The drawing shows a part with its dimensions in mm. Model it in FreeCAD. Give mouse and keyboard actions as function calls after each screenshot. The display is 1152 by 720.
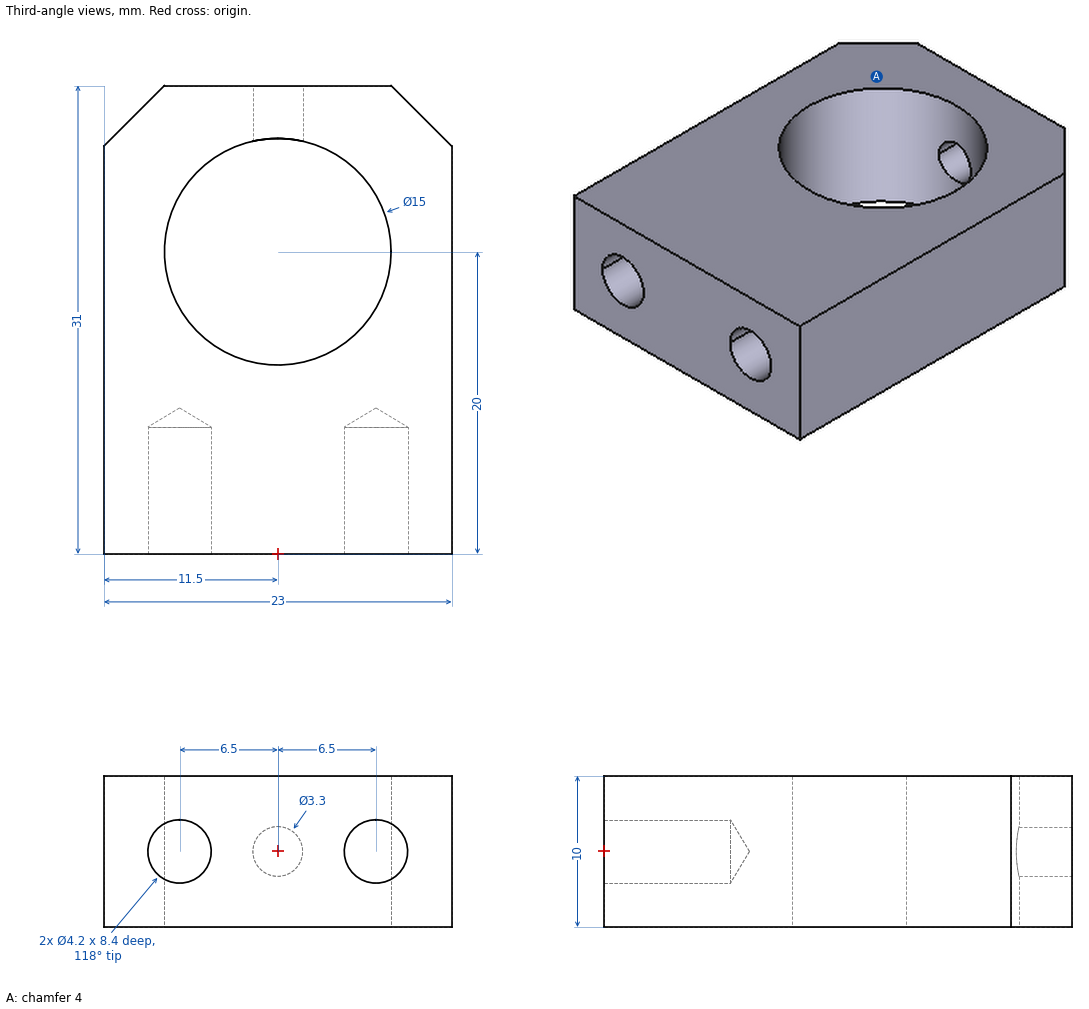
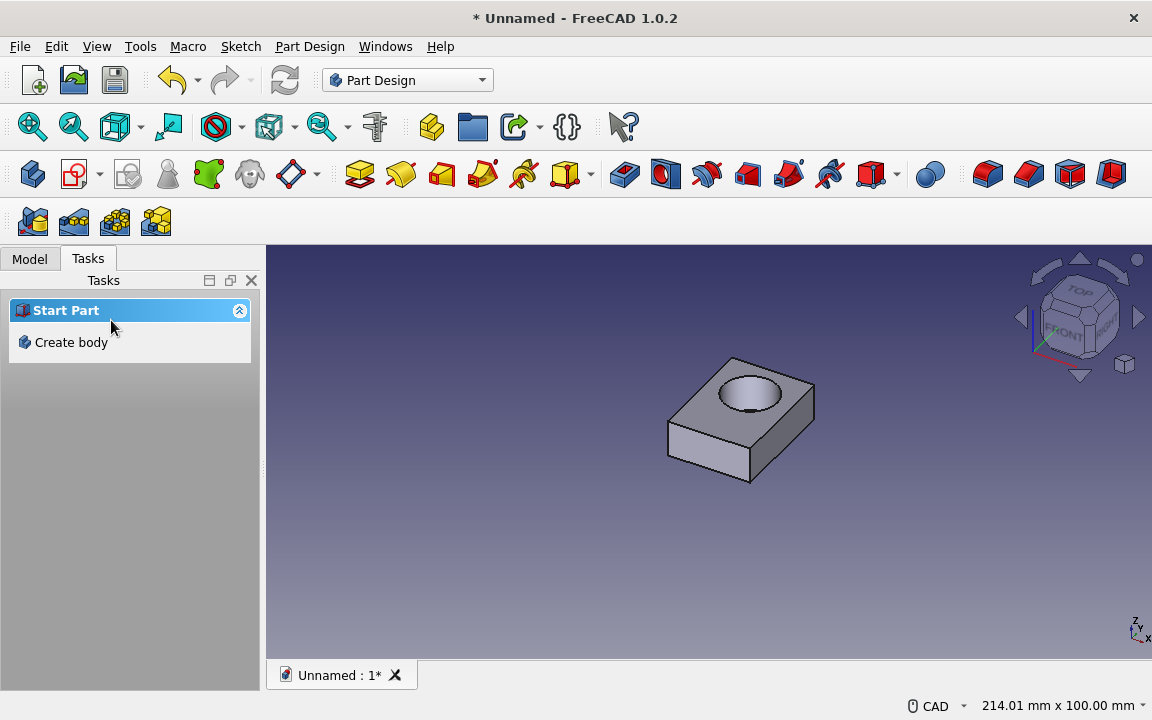
click(33, 128)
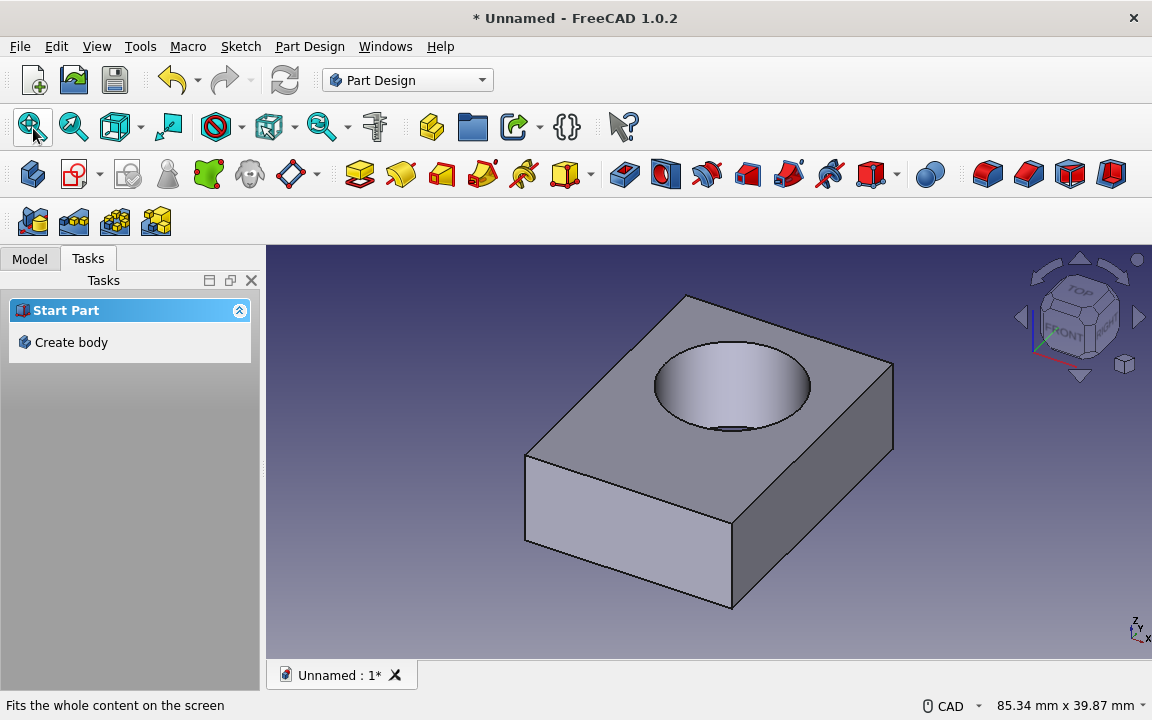
key(0)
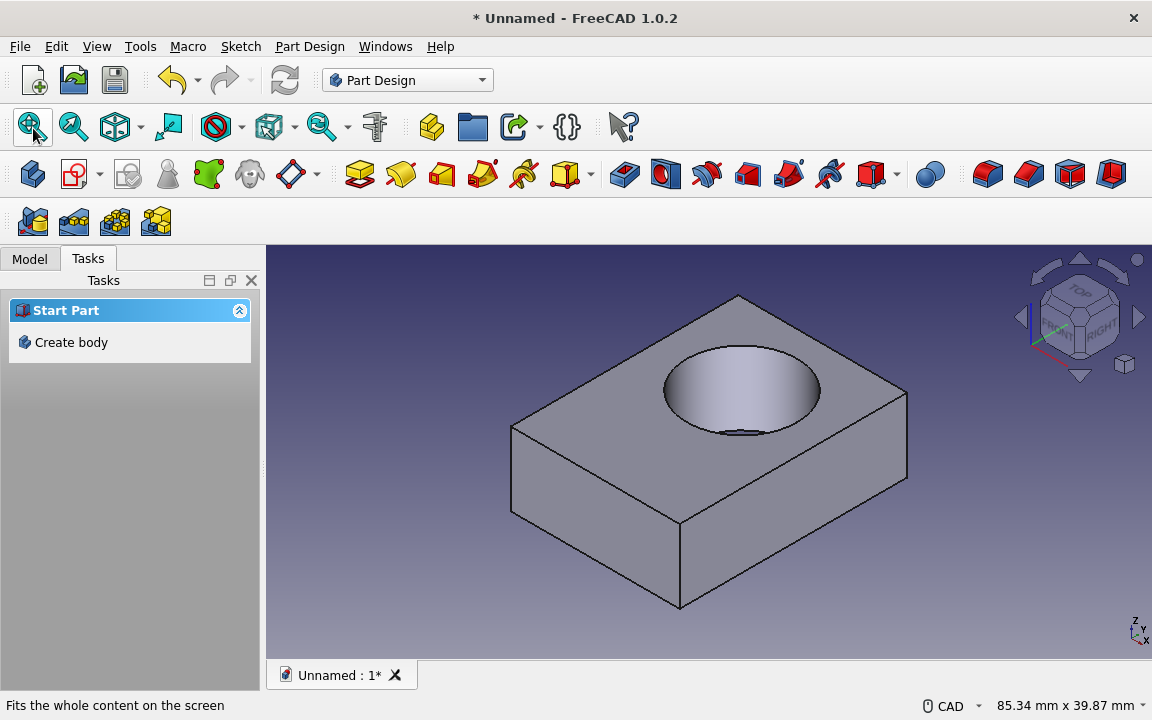
key(2)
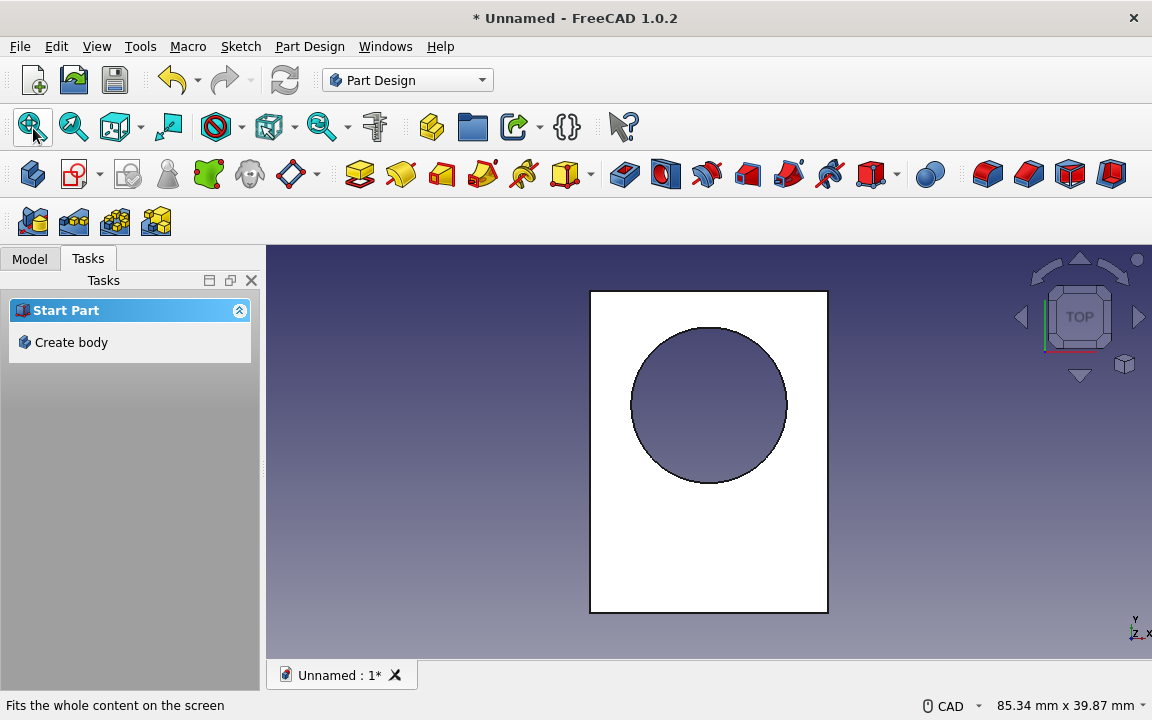
key(1)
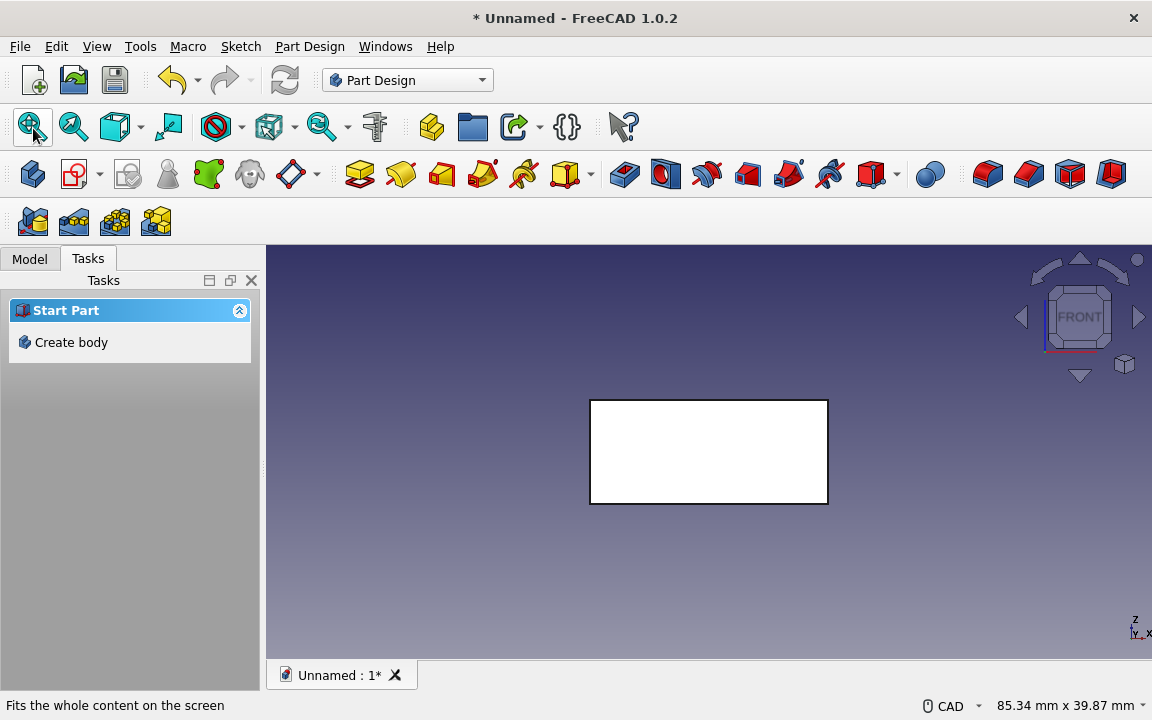
key(v)
key(f)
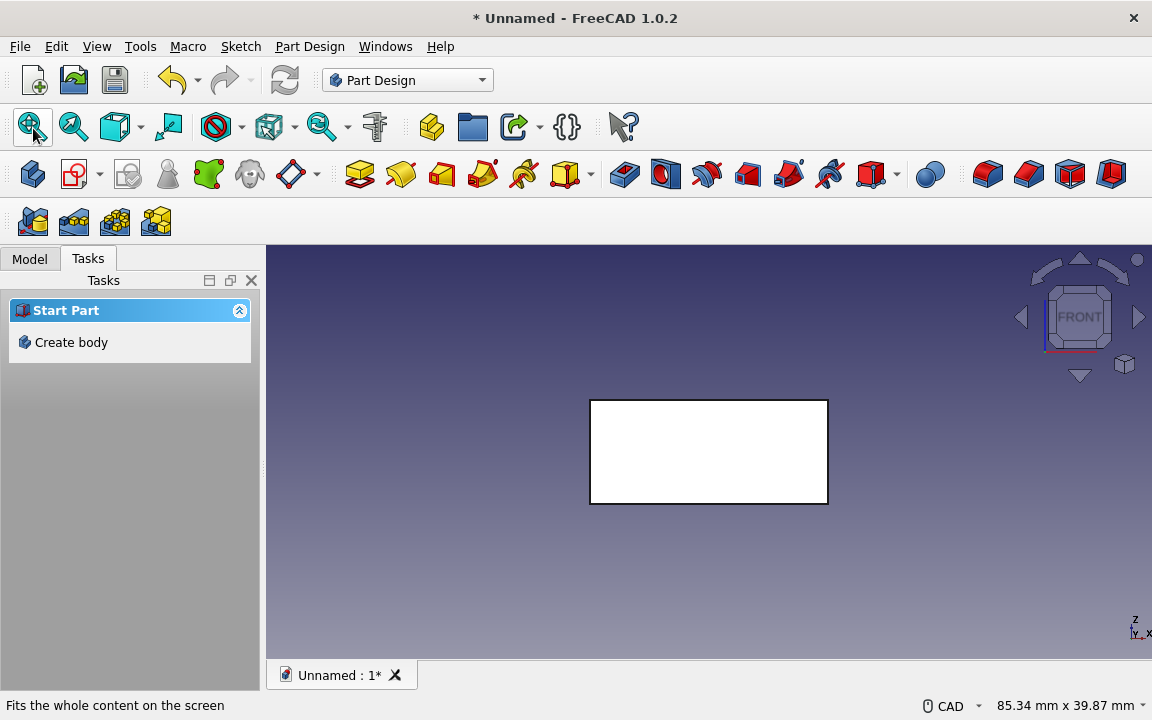
key(3)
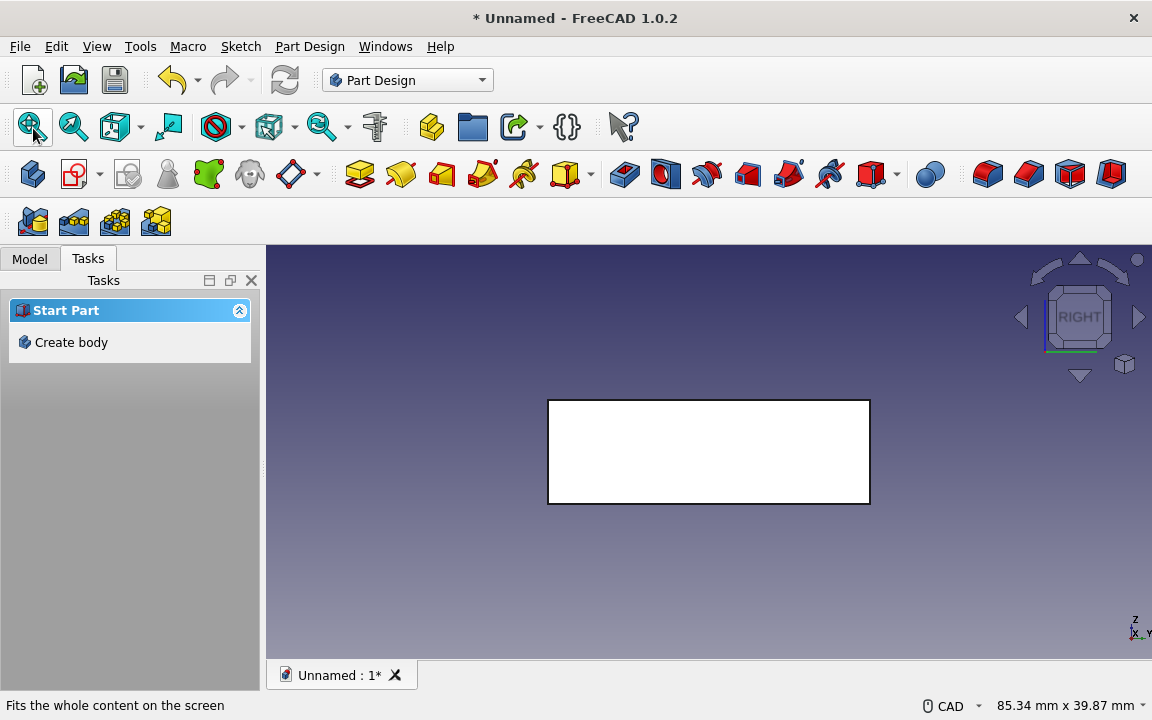
key(v)
key(f)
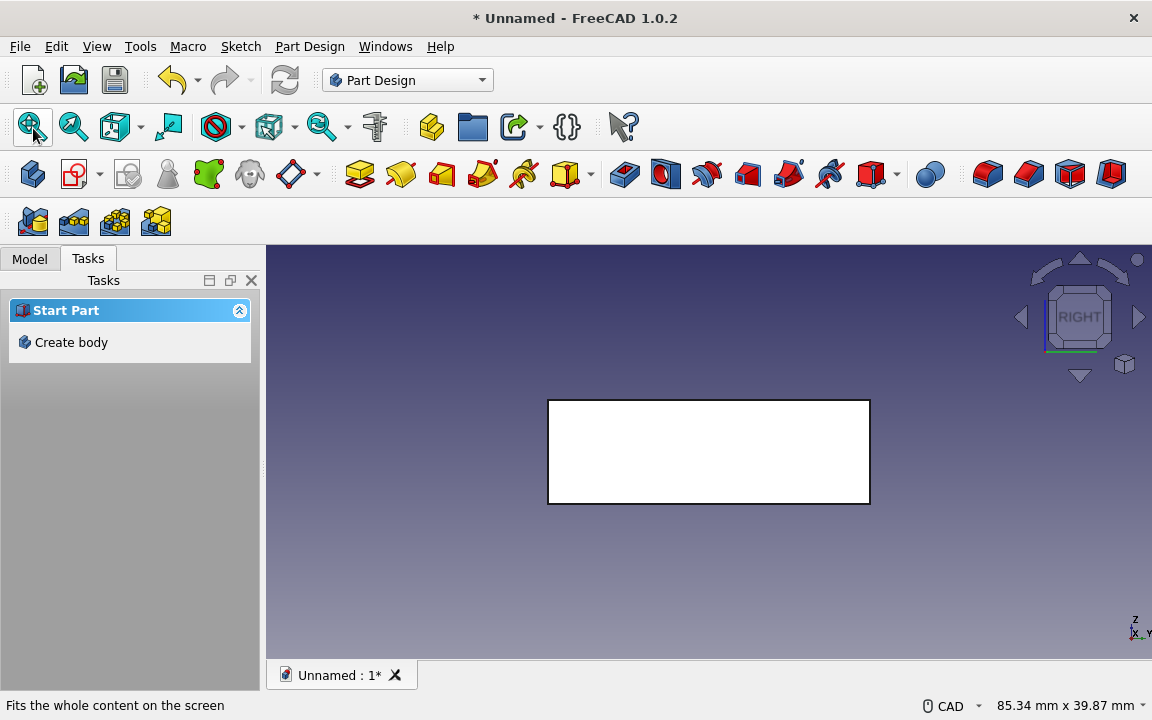
click(870, 451)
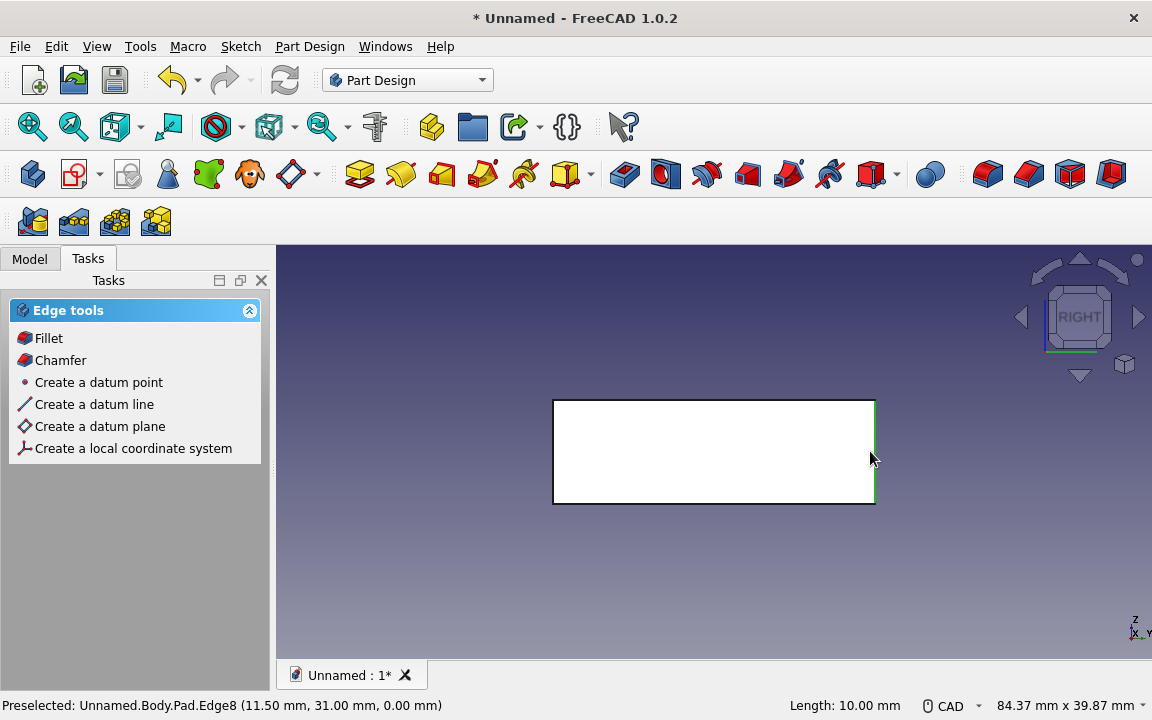
key(5)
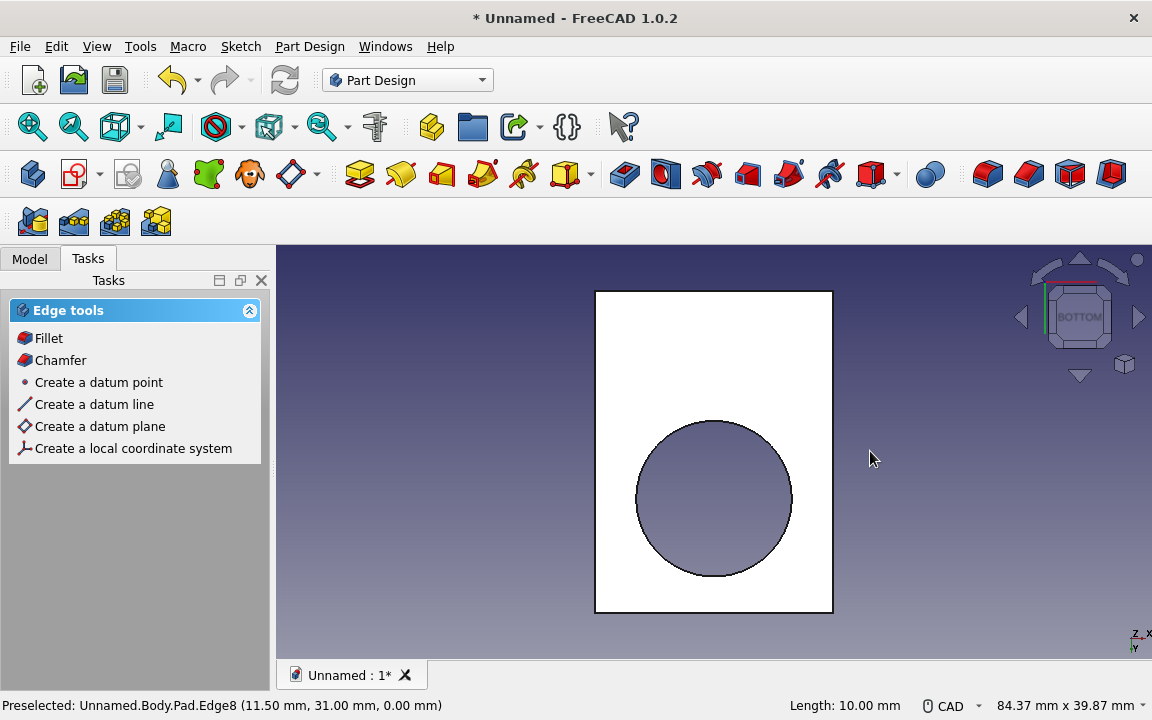
key(4)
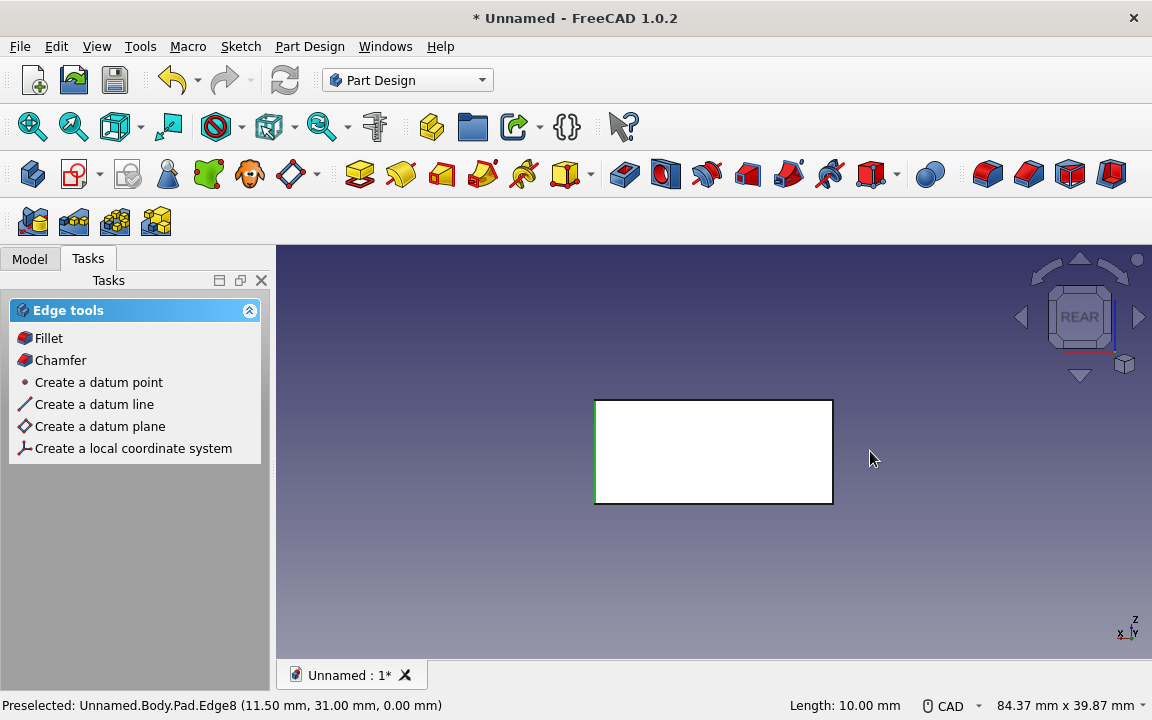
key(v)
key(f)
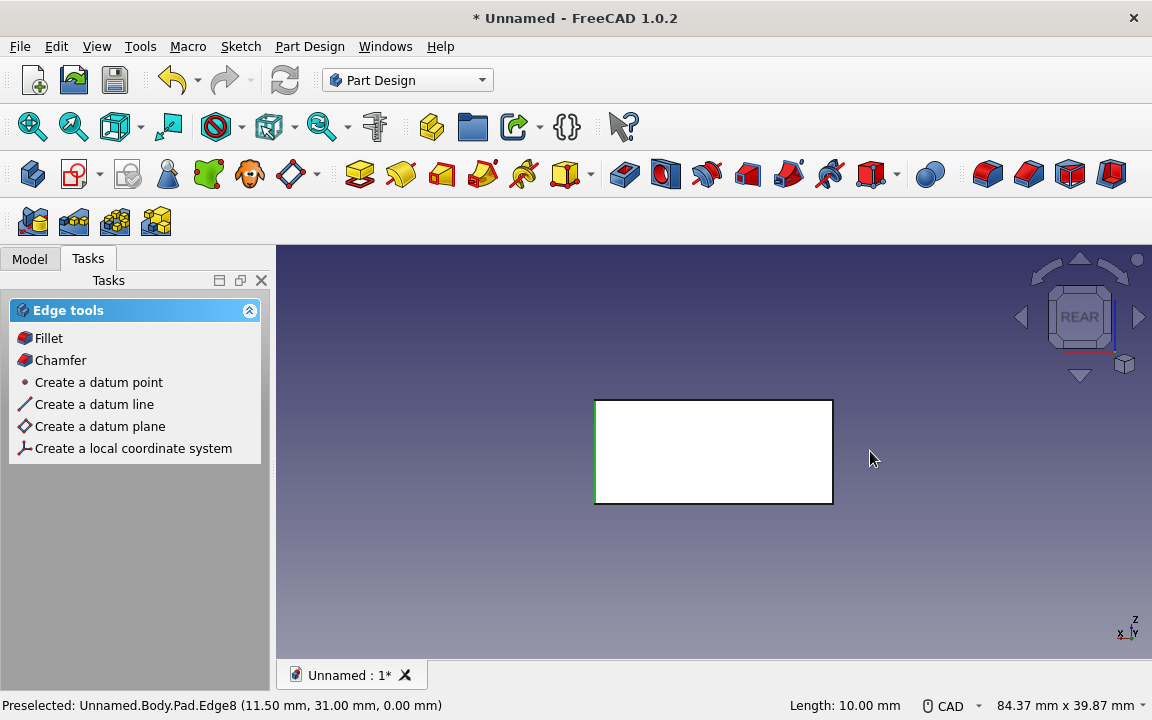
click(833, 451, ctrl)